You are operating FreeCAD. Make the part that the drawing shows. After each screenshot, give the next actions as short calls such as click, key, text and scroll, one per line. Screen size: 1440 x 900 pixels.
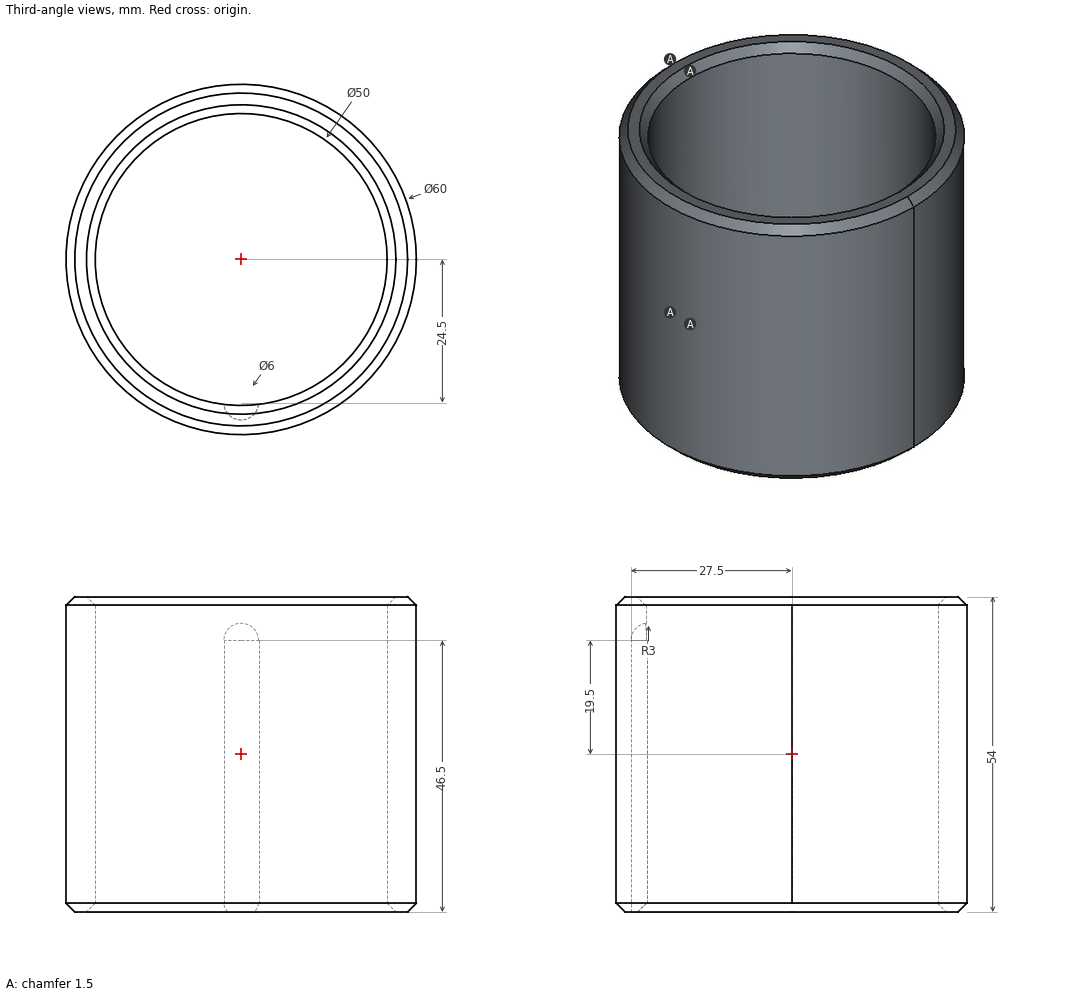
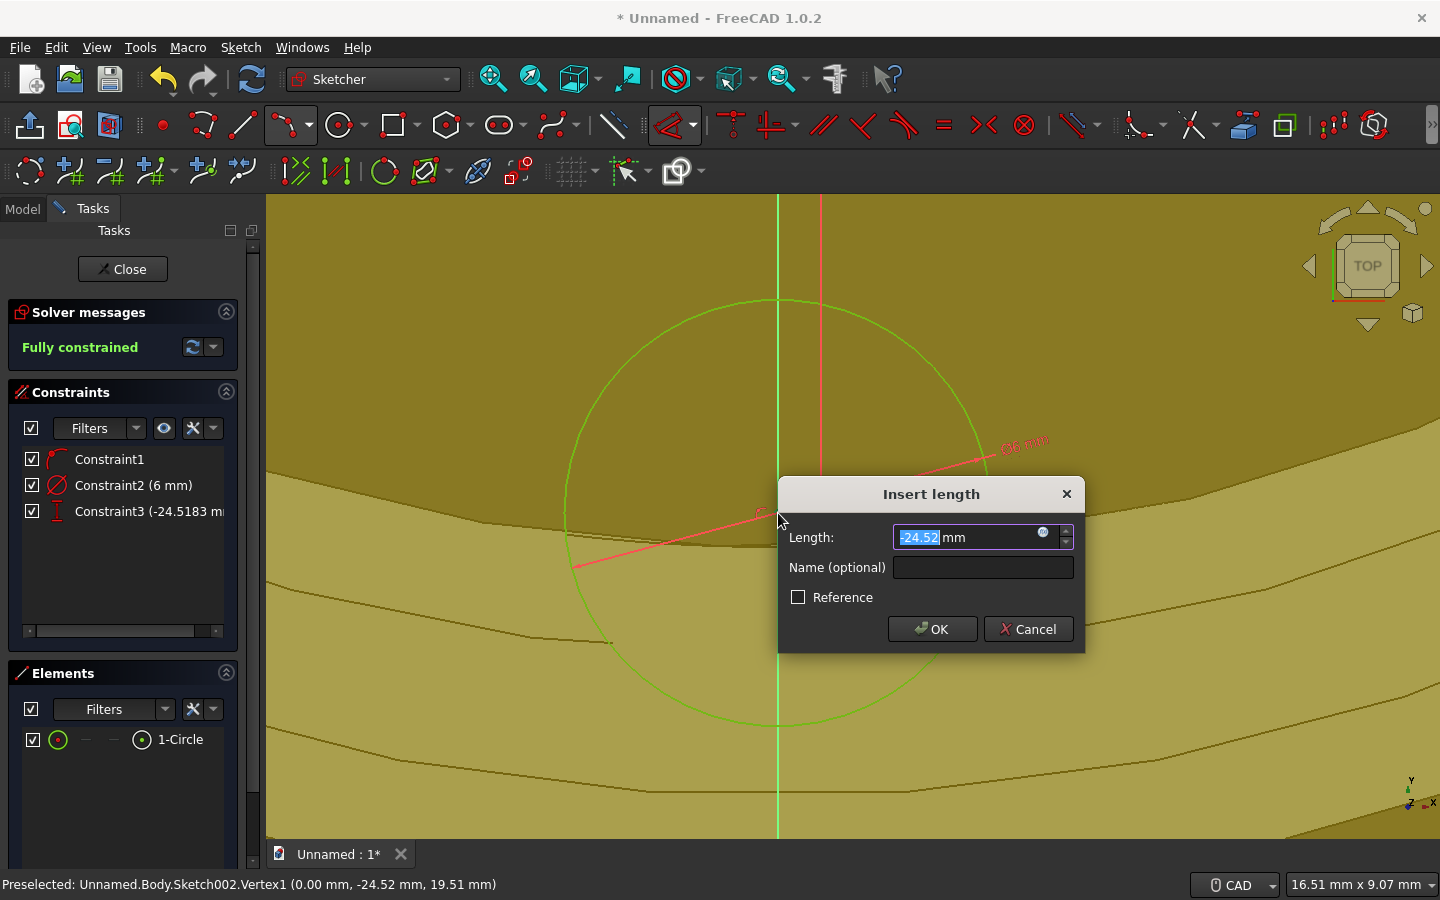
text(-24.5)
key(Return)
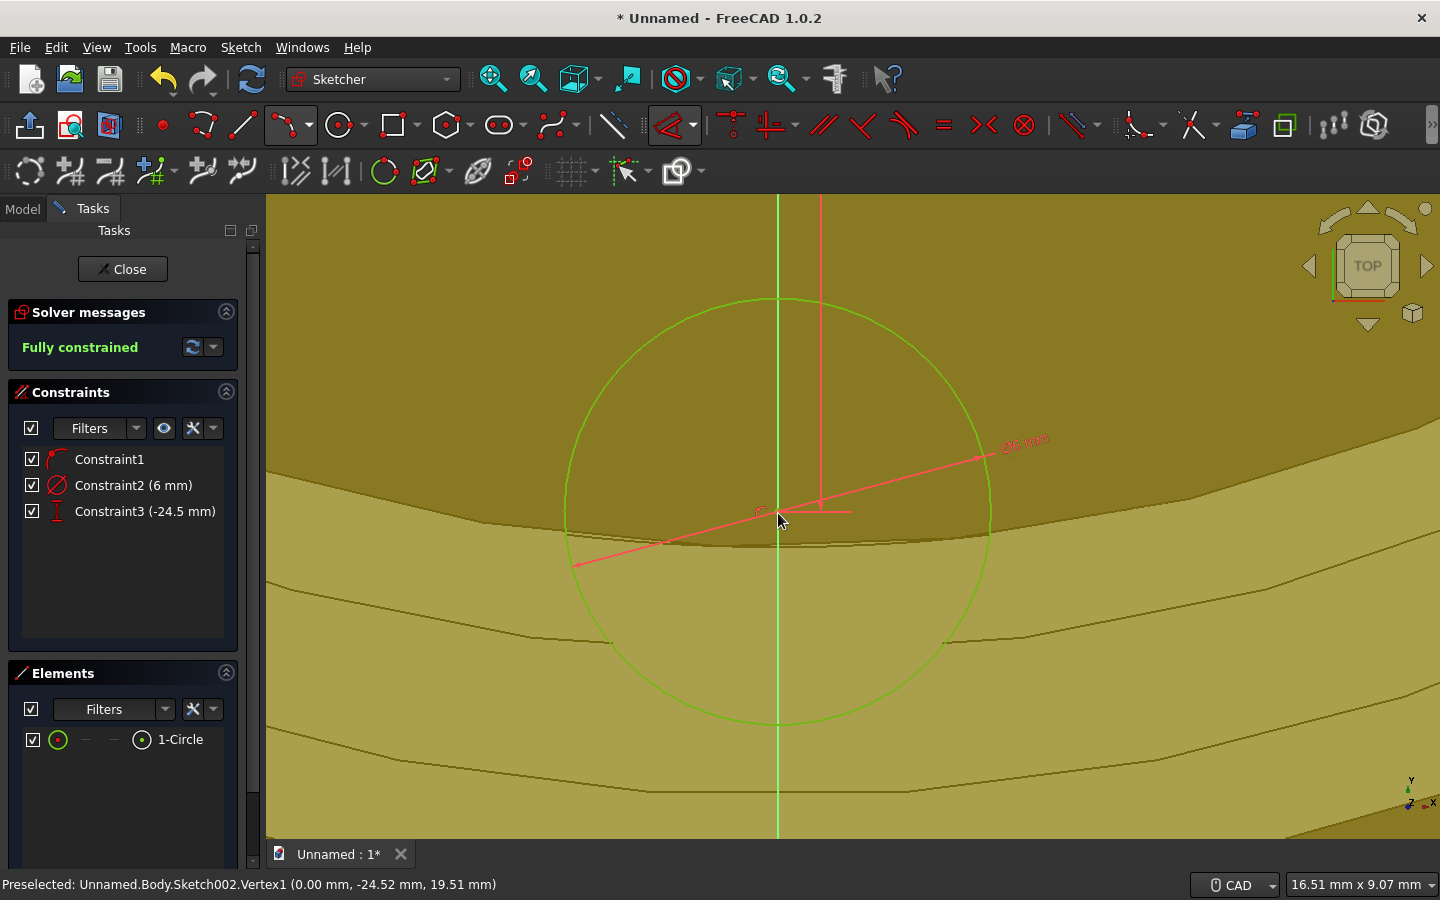
click(123, 269)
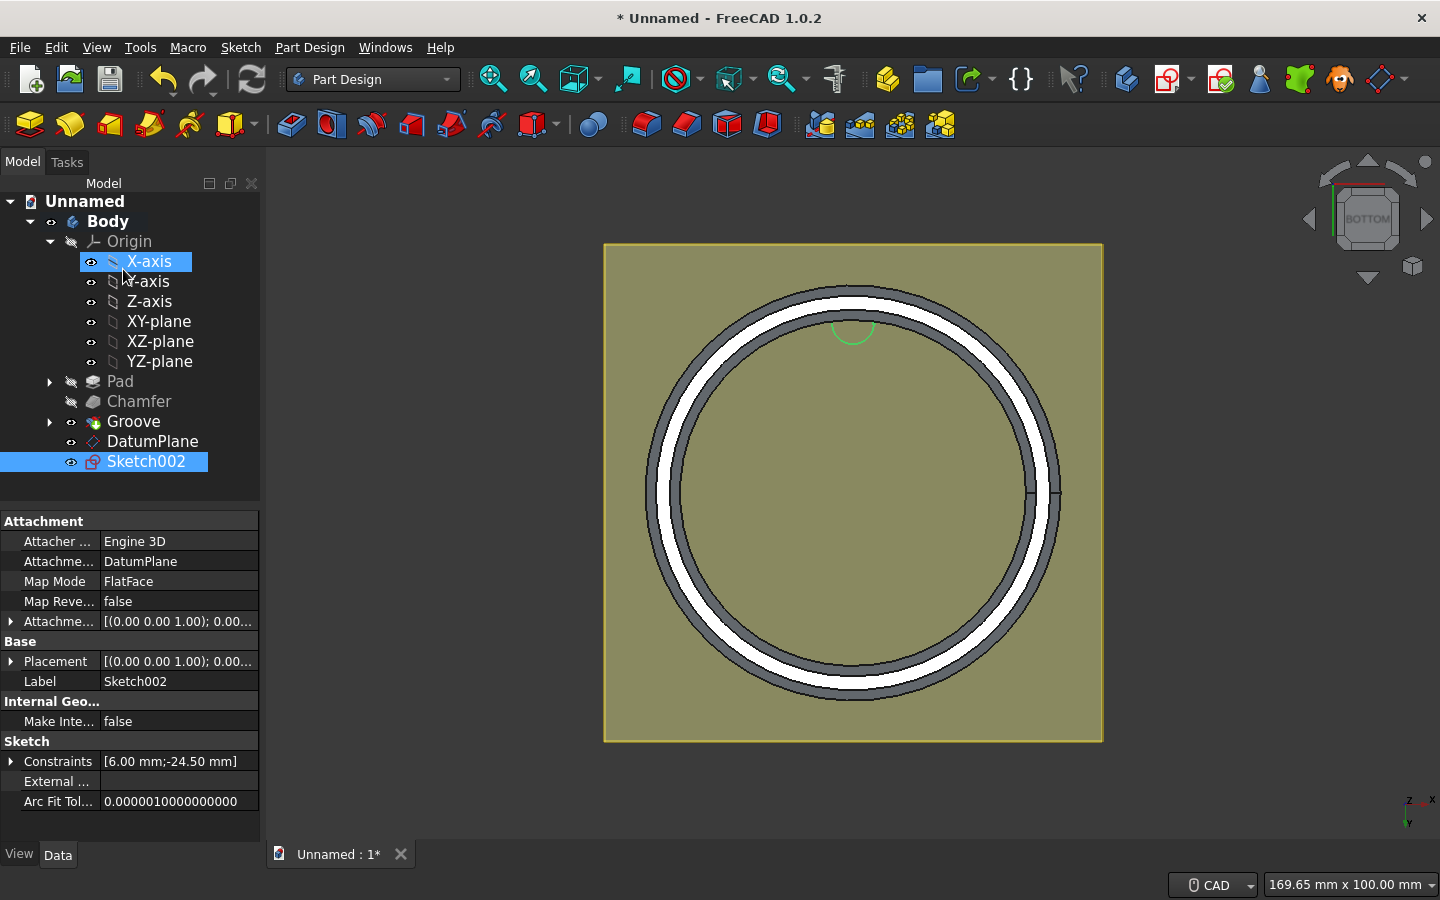
click(292, 124)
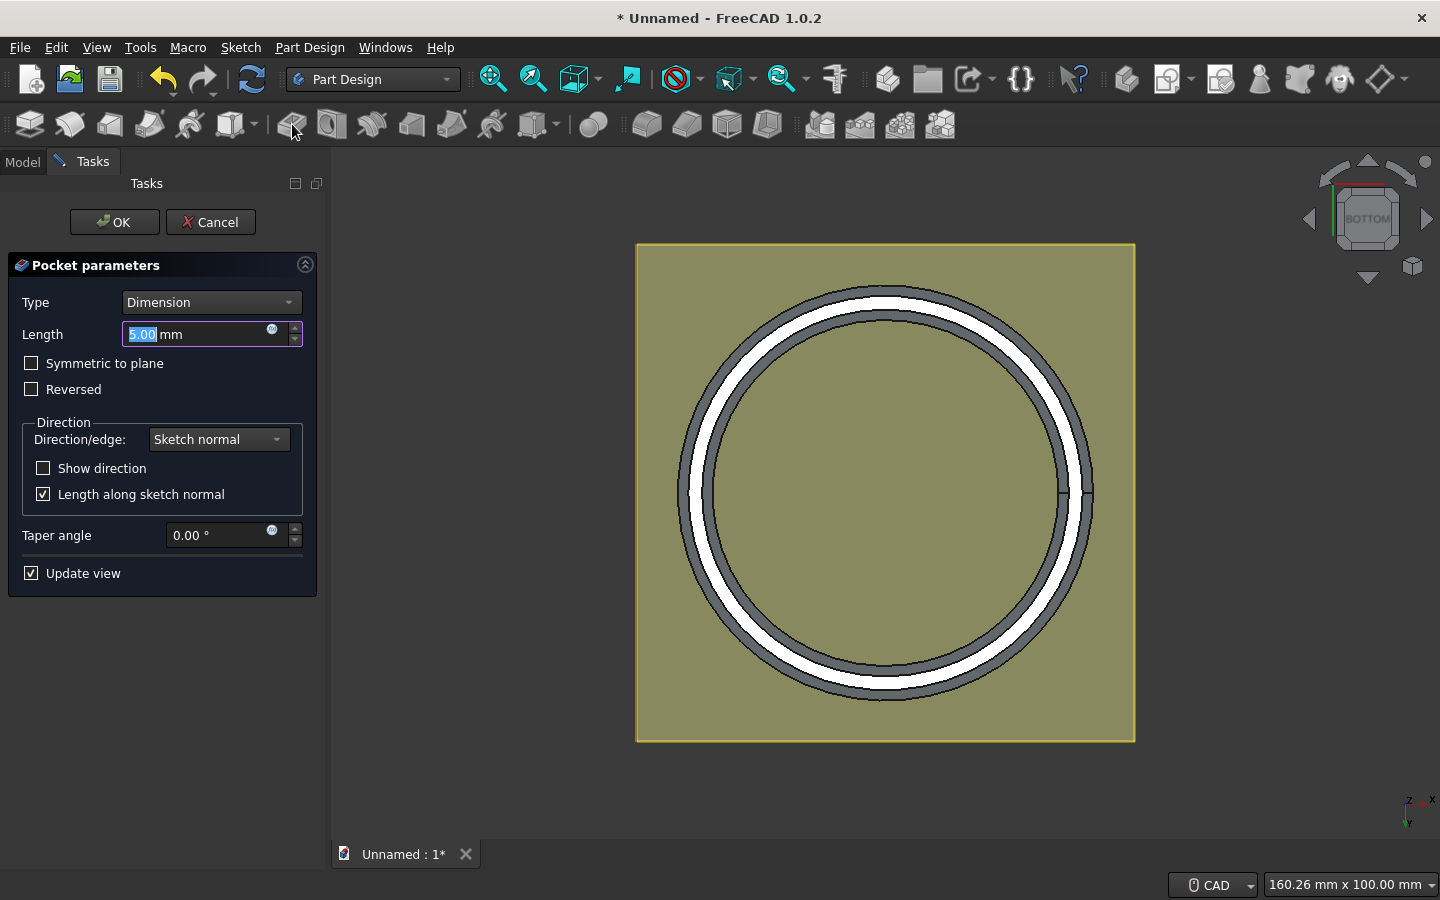
text(46.5)
key(Tab)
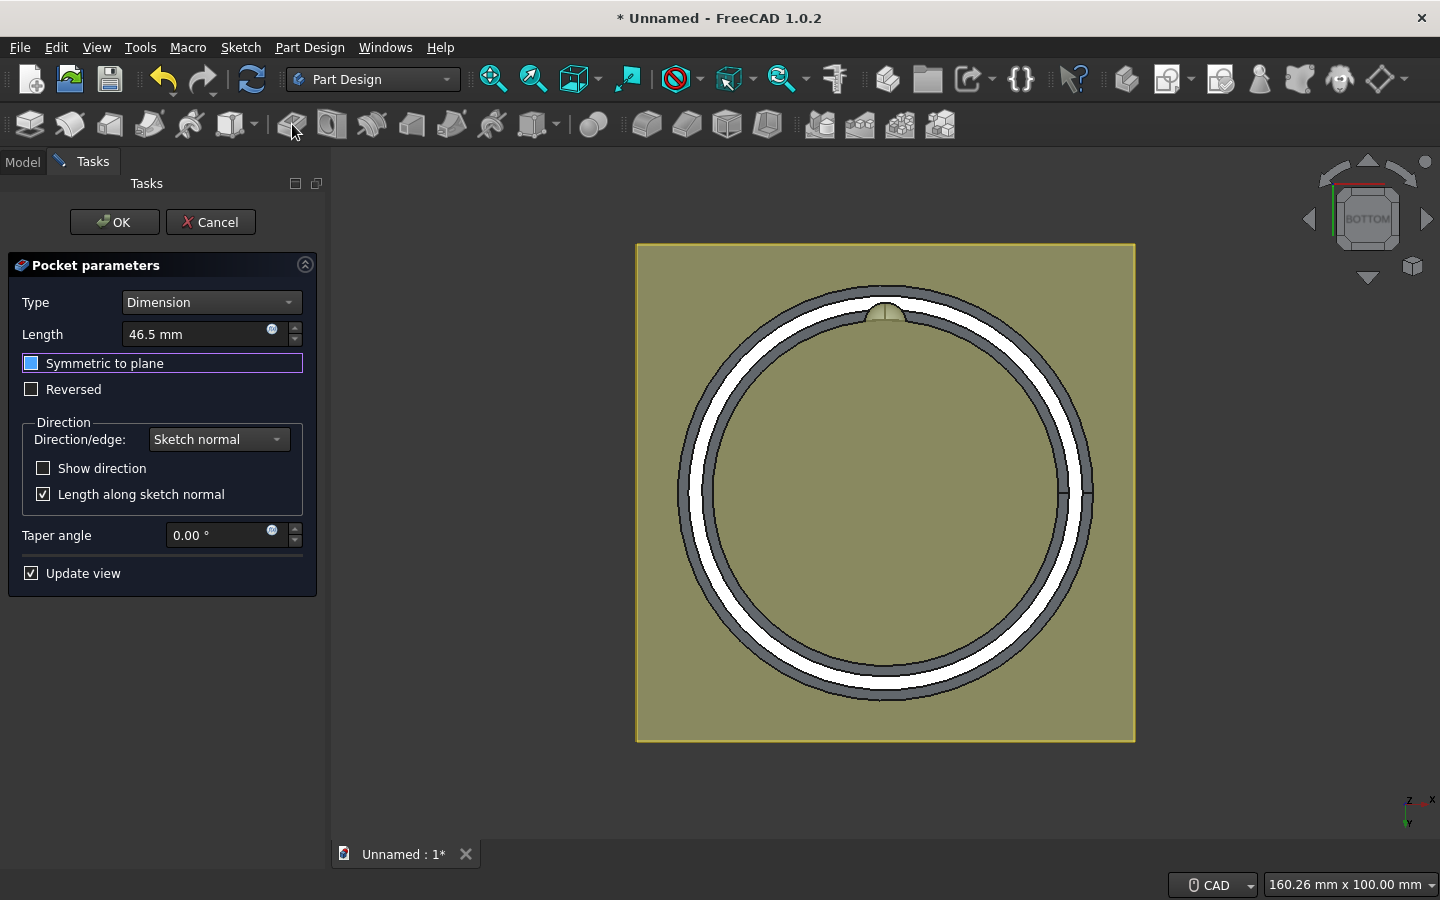
click(115, 222)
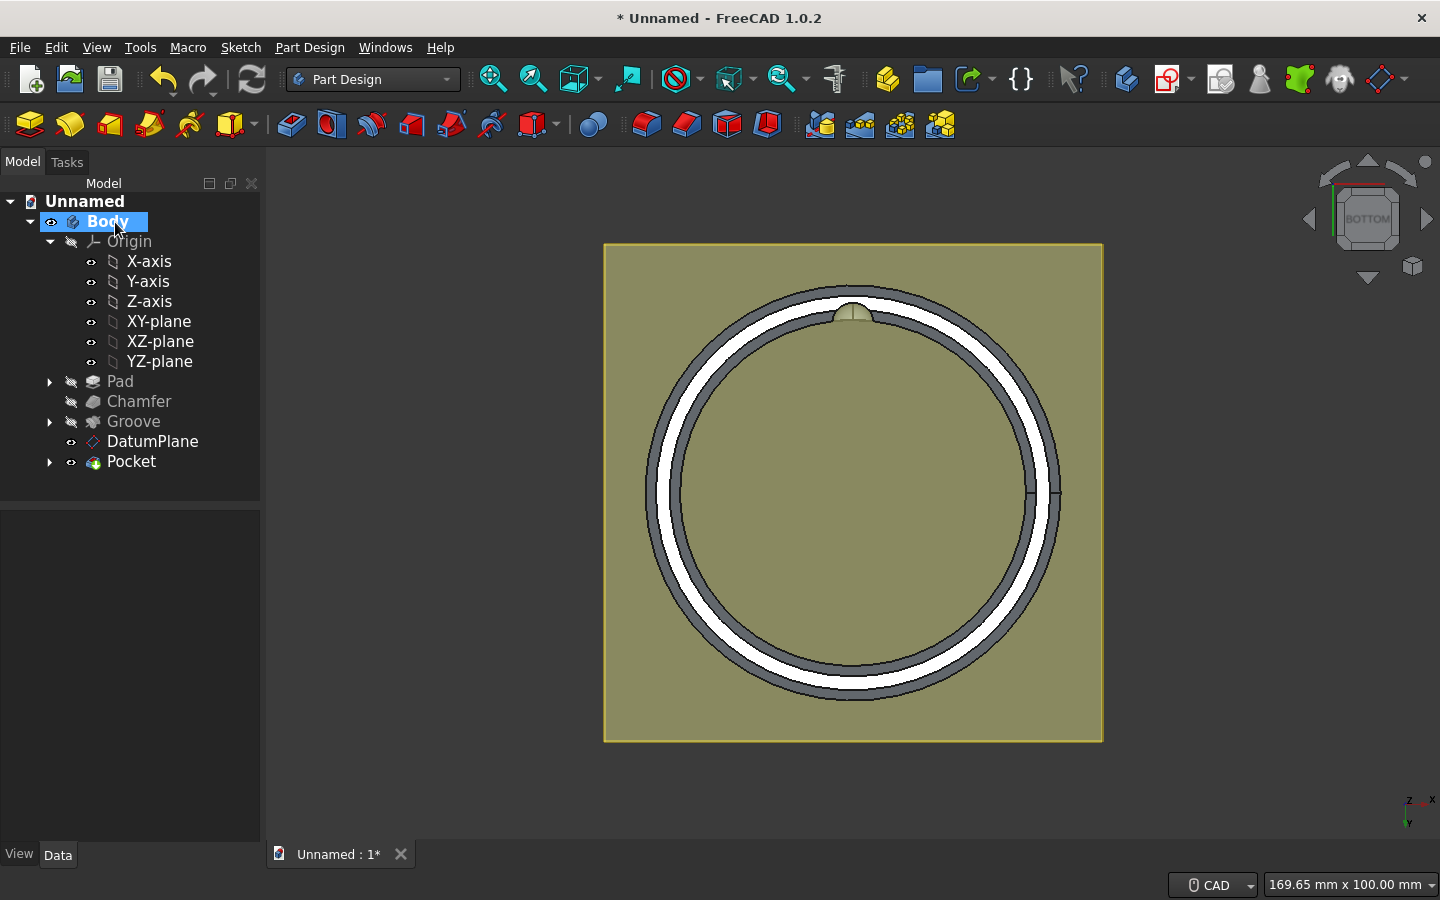
click(116, 442)
key(space)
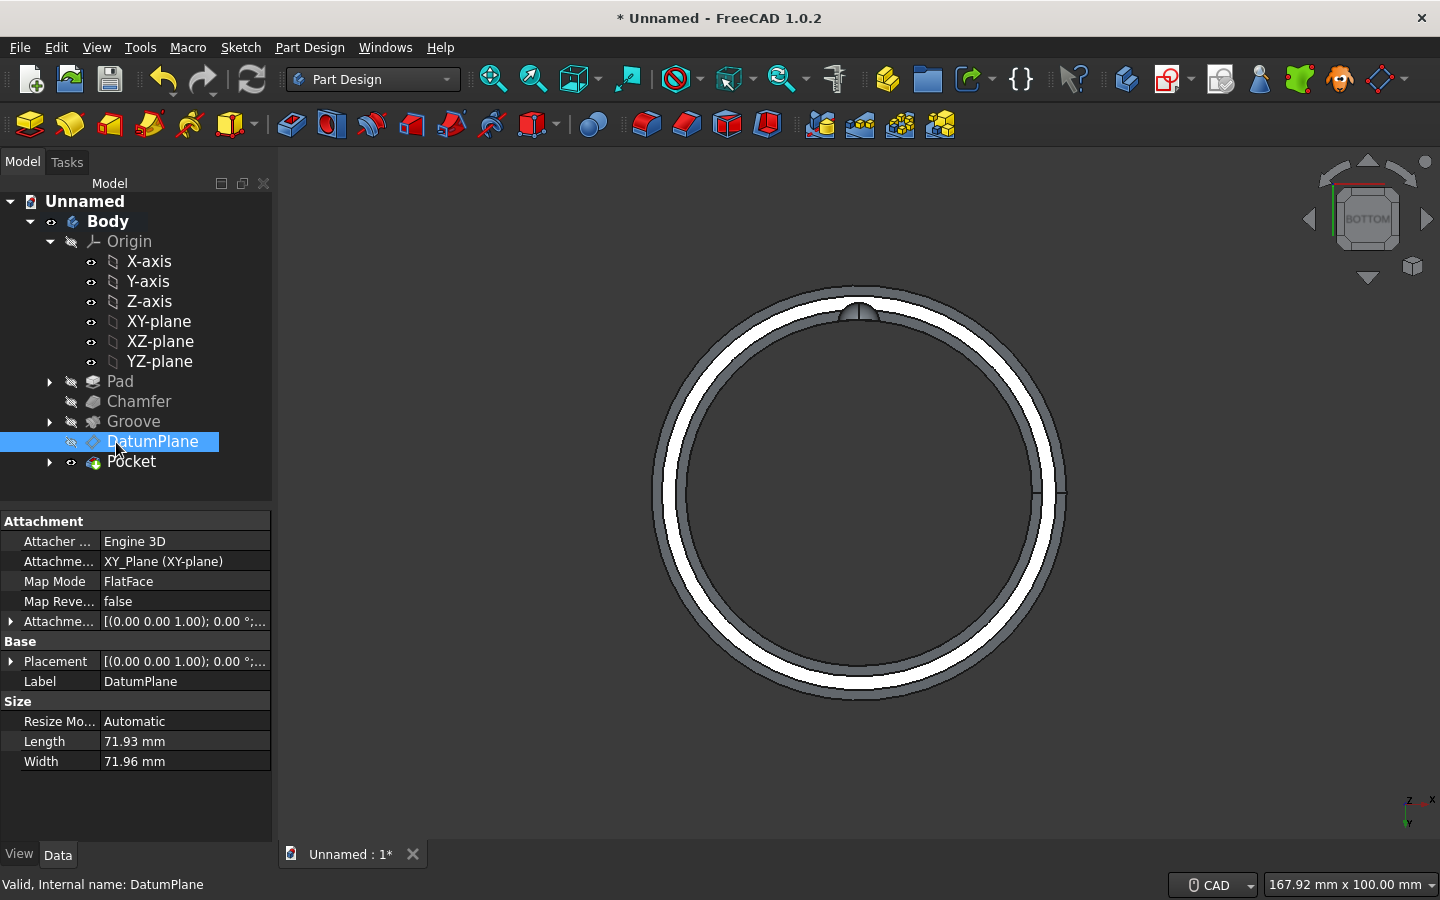
key(0)